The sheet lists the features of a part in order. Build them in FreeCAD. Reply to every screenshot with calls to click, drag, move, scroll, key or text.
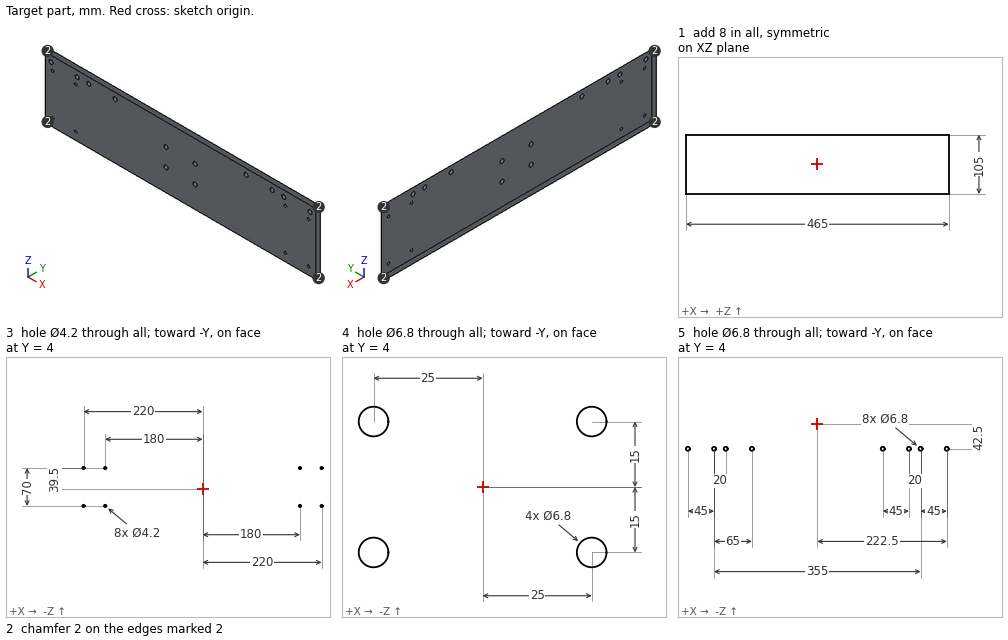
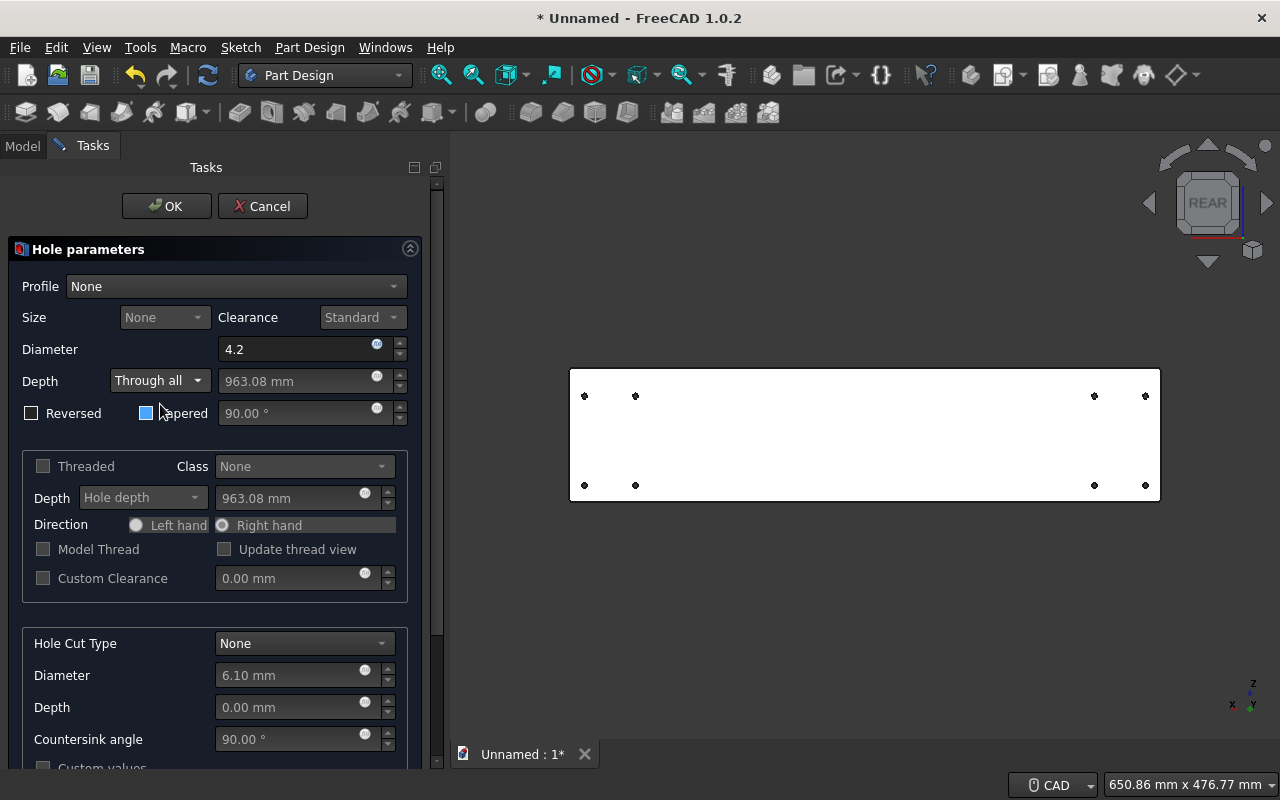
click(167, 206)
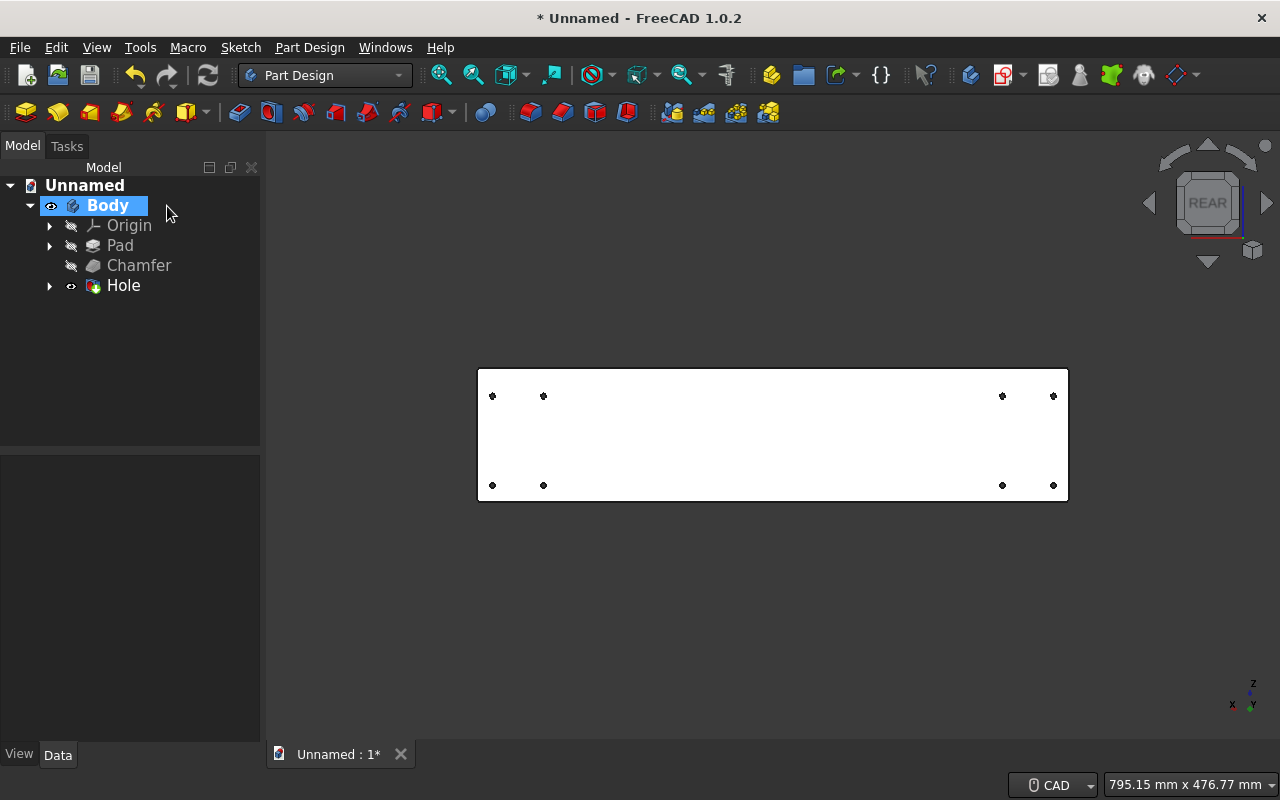
click(604, 434)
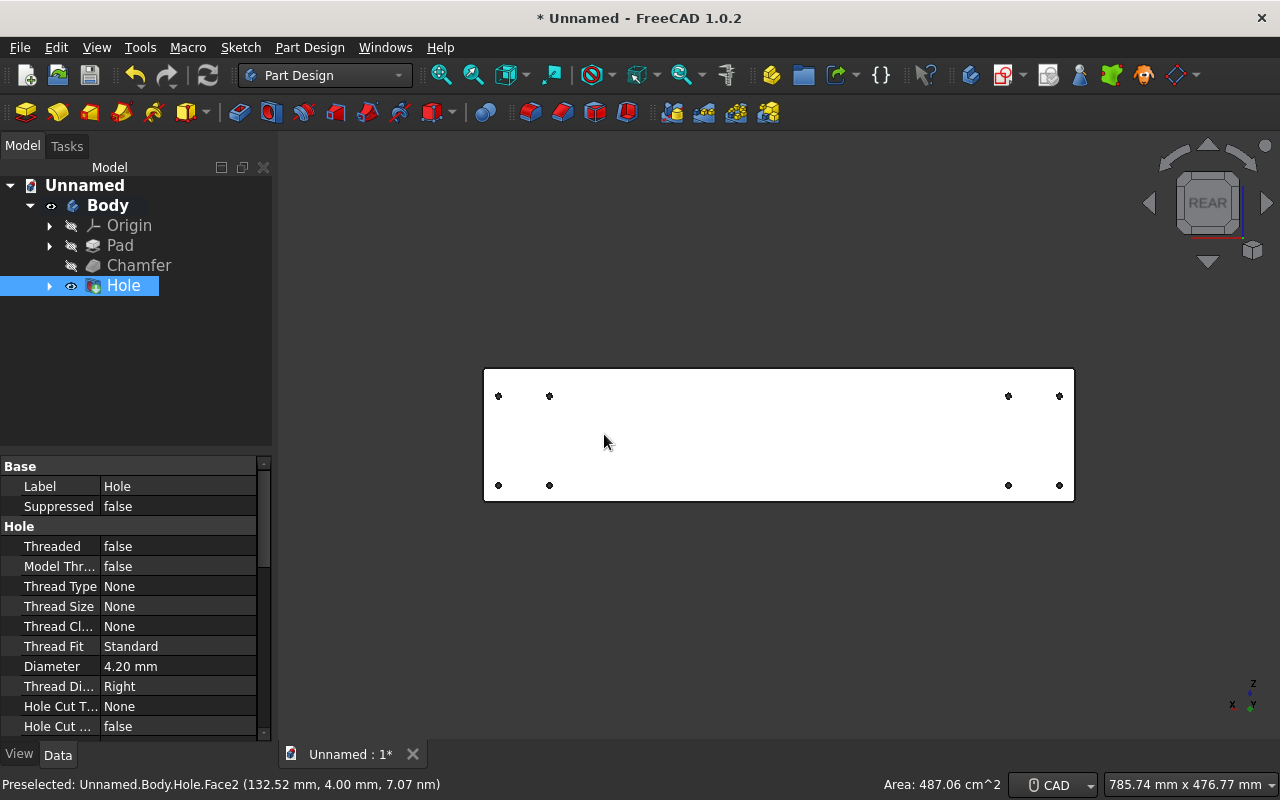
click(1004, 76)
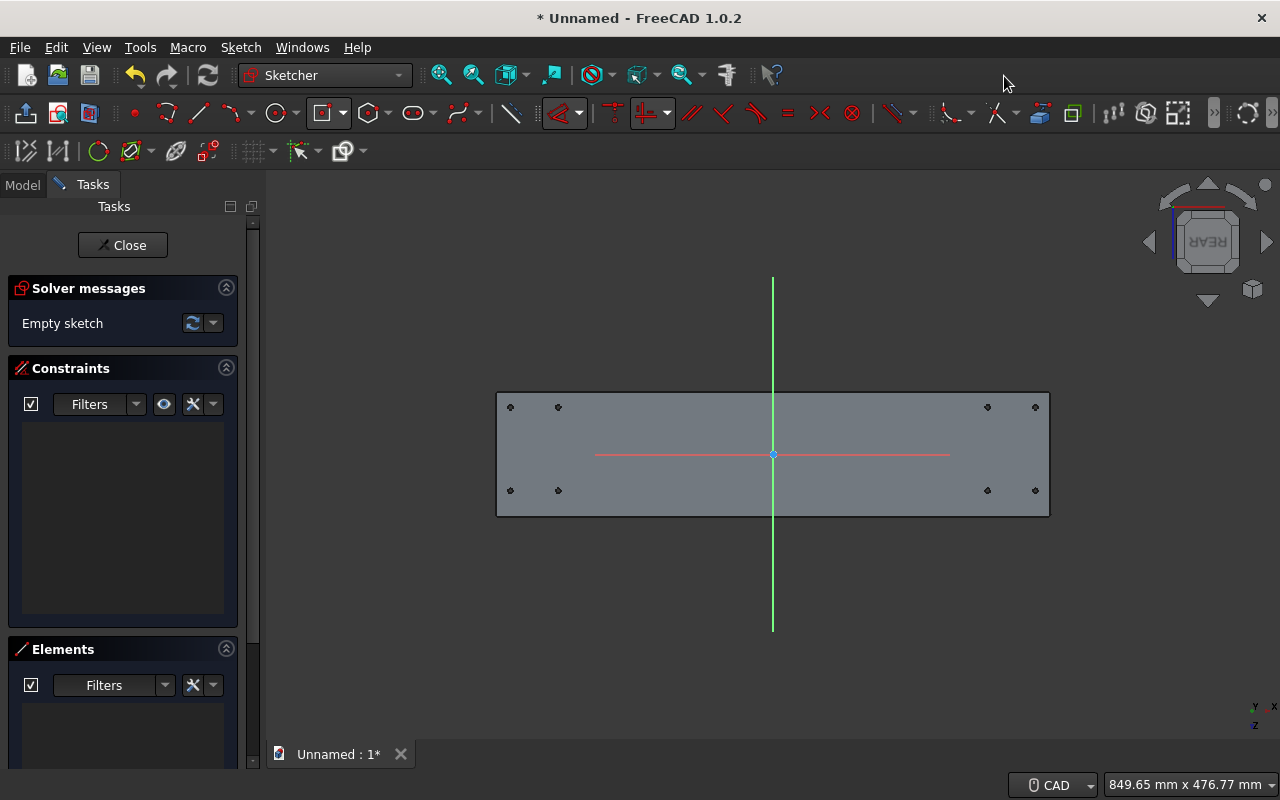
scroll(782, 454, up, 11)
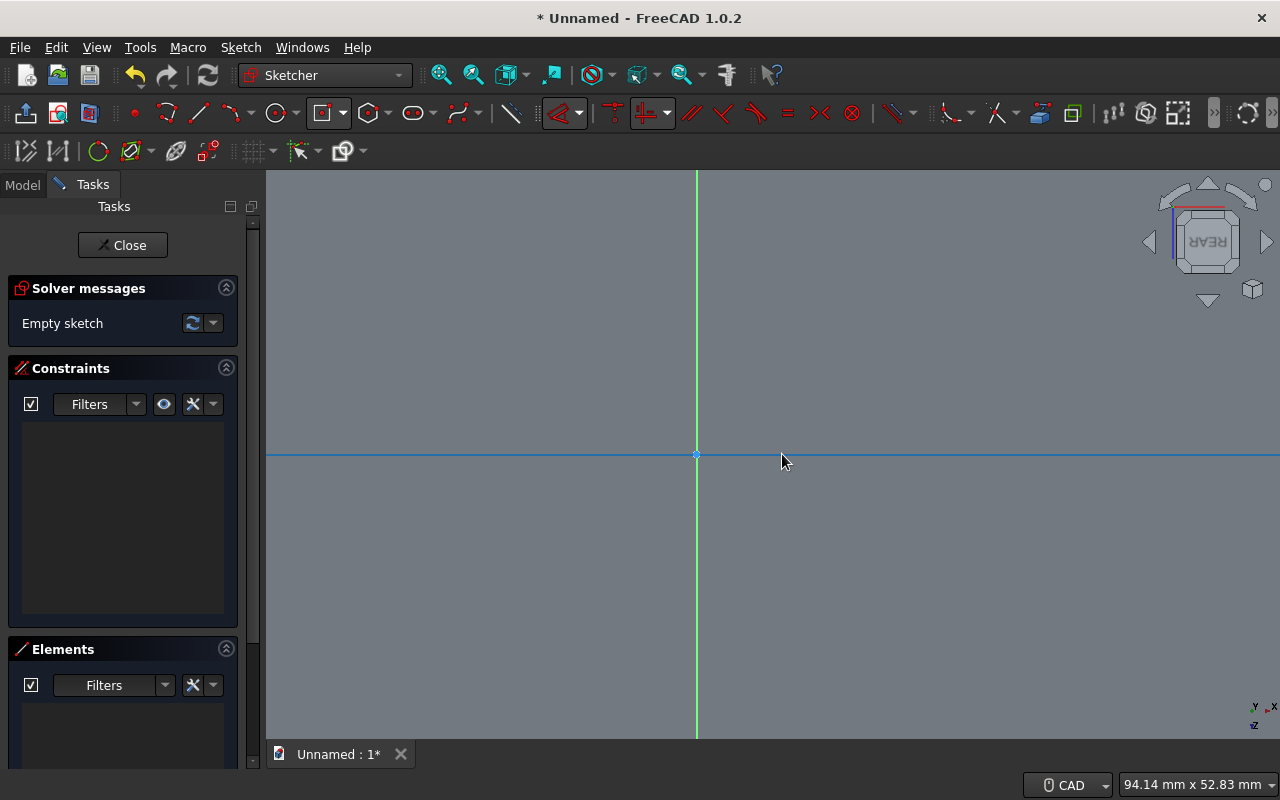
click(276, 114)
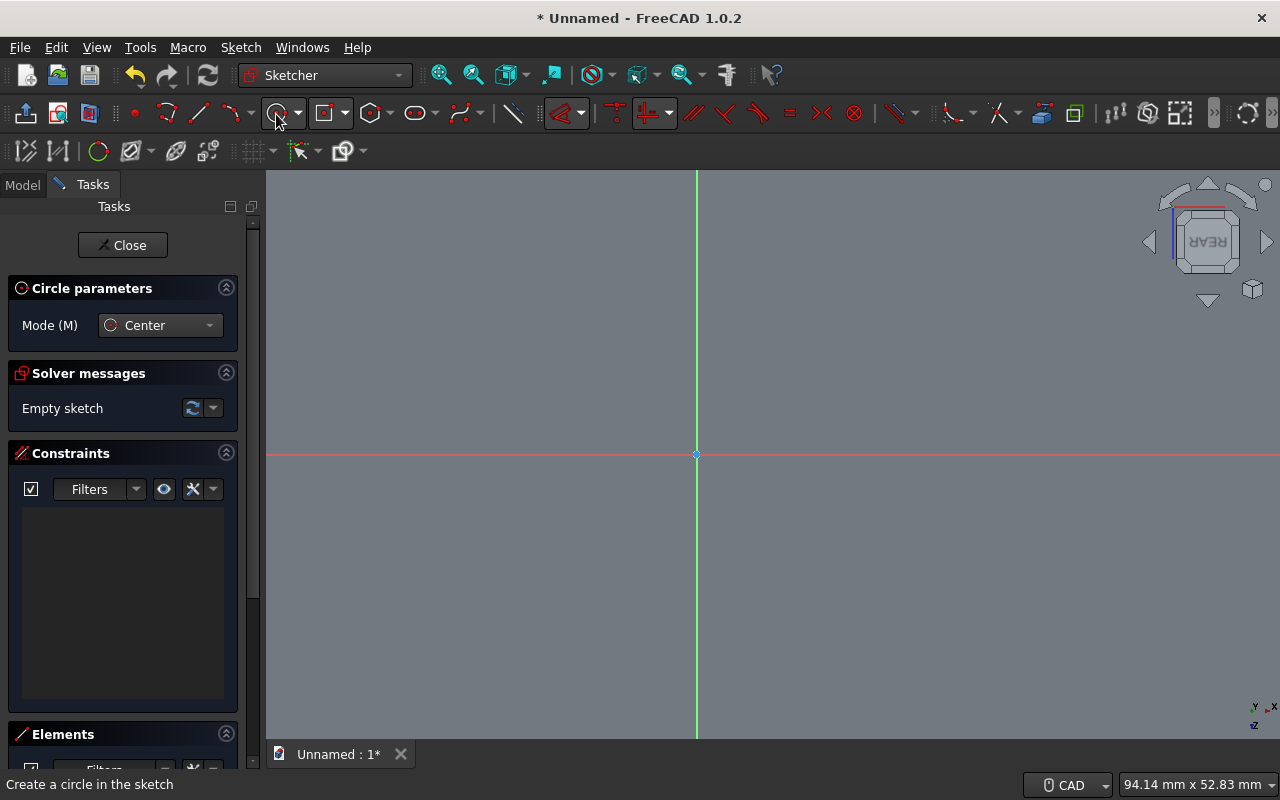
click(966, 616)
move(992, 590)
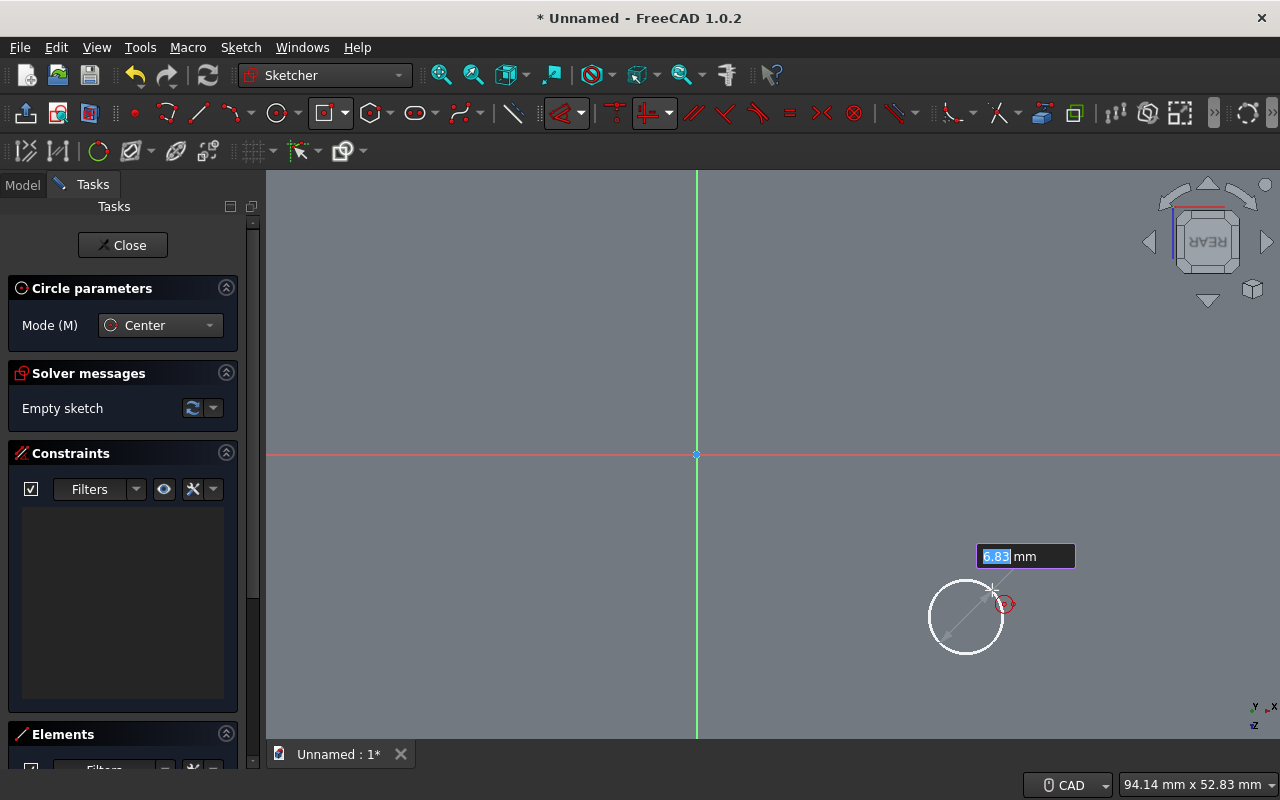
text(6.8)
key(Return)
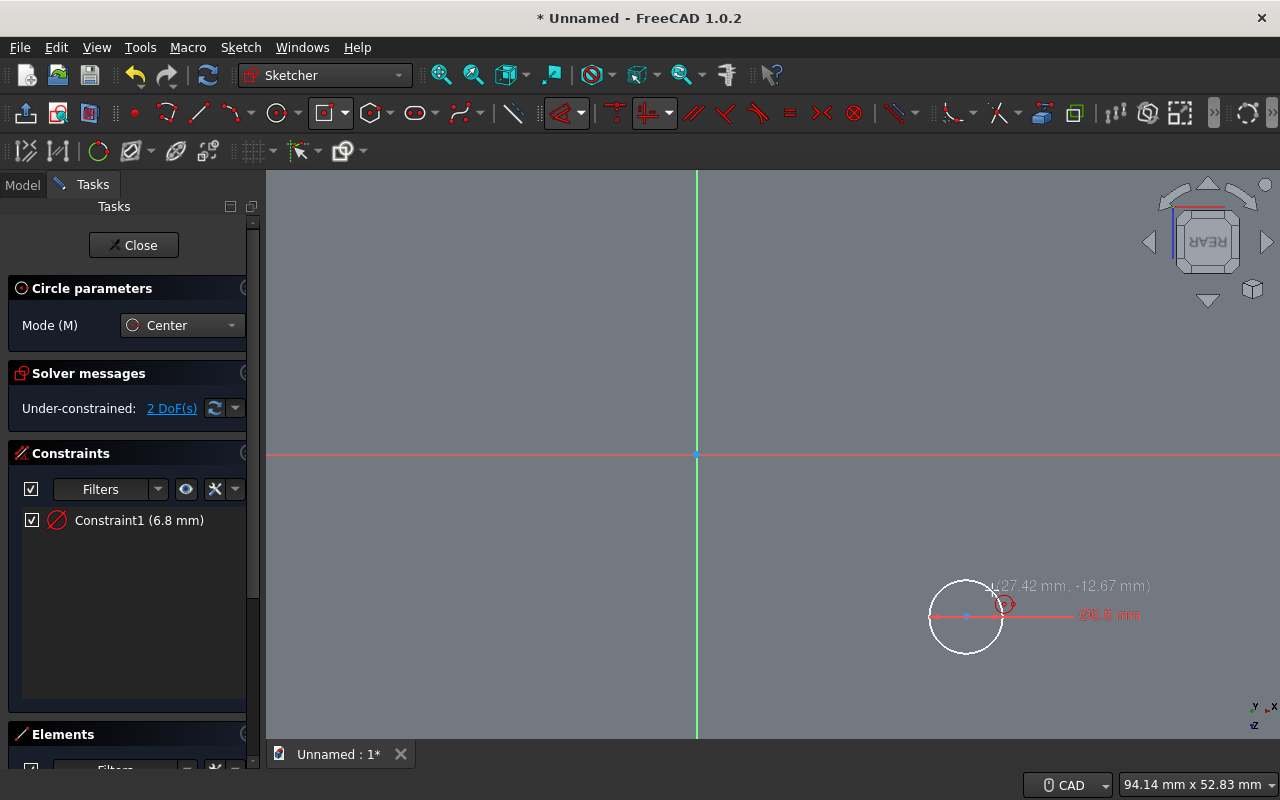
click(966, 293)
move(992, 267)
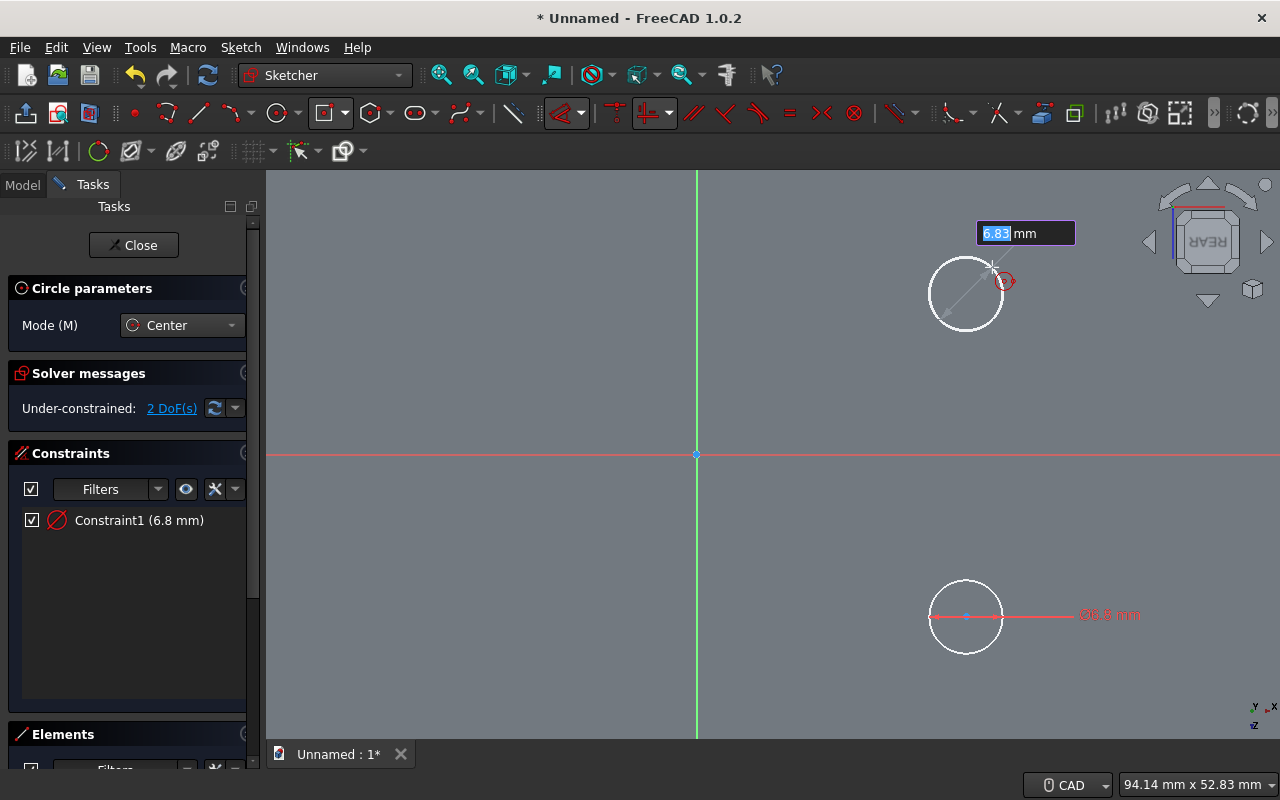
text(6.8)
key(Return)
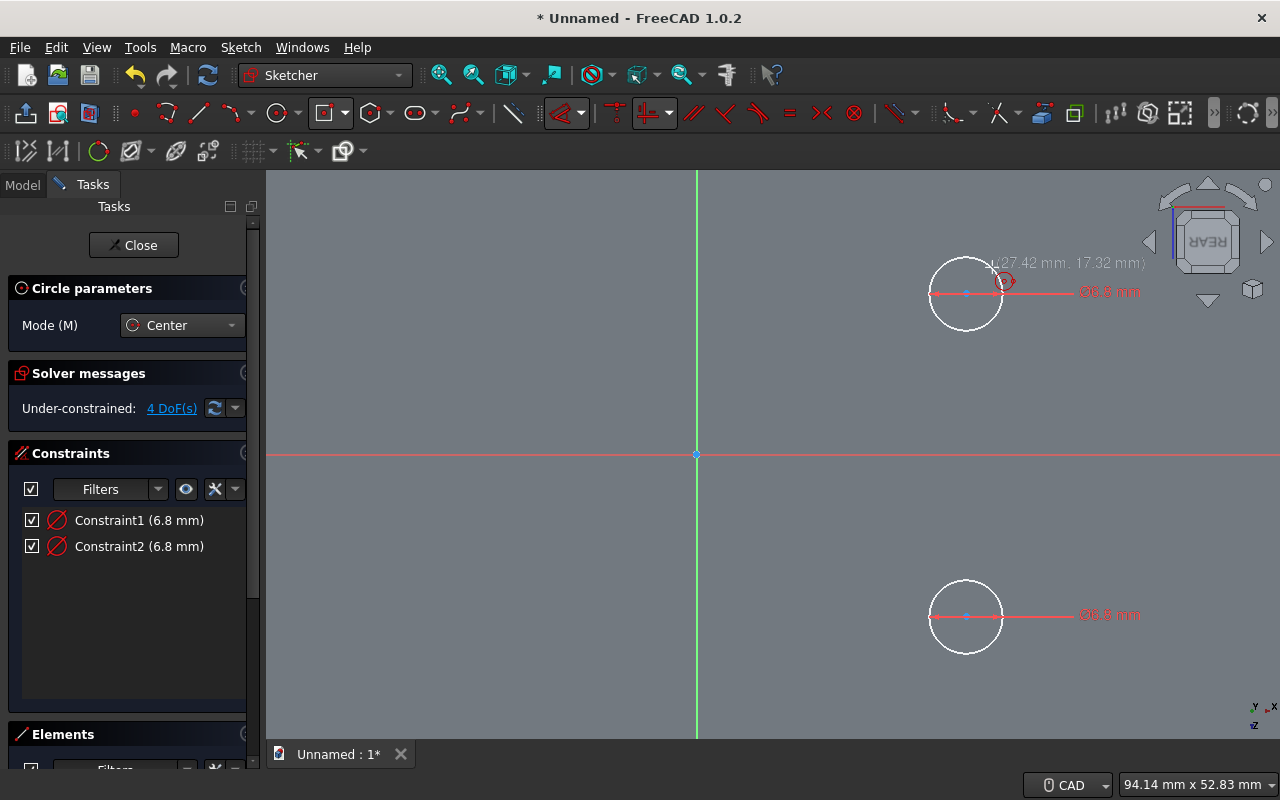
click(427, 293)
move(453, 267)